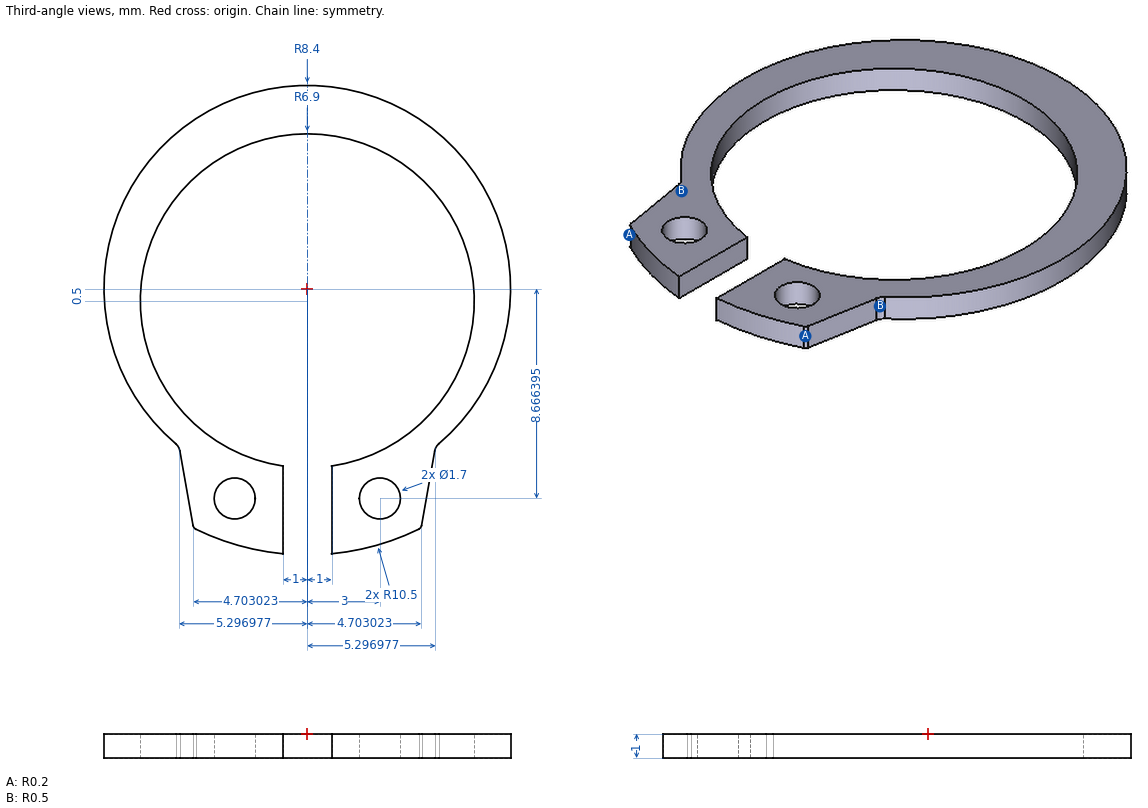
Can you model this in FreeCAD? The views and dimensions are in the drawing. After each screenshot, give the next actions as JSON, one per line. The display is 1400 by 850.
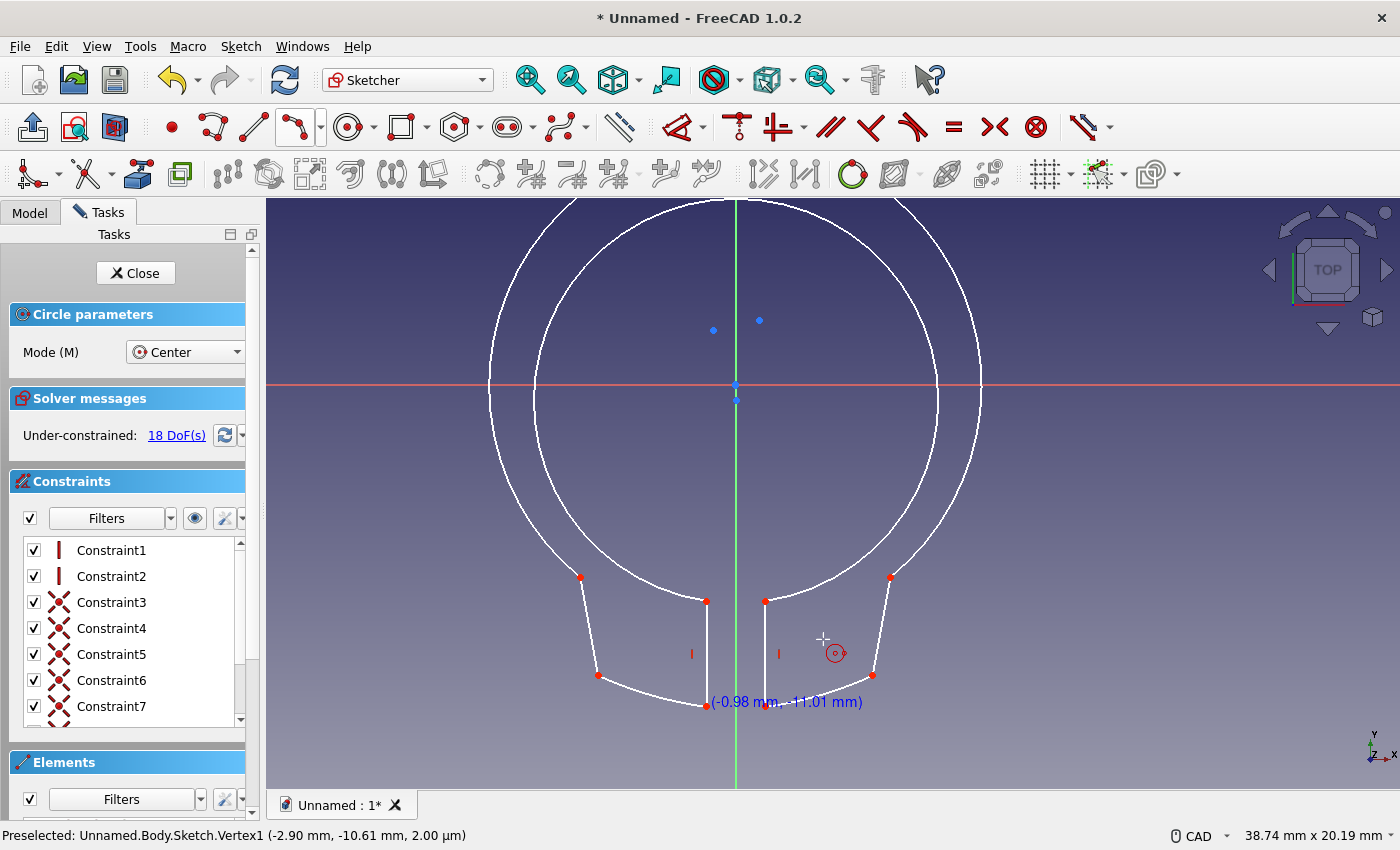
{"action": "left_click", "coordinate": [823, 638]}
{"action": "left_click", "coordinate": [841, 621]}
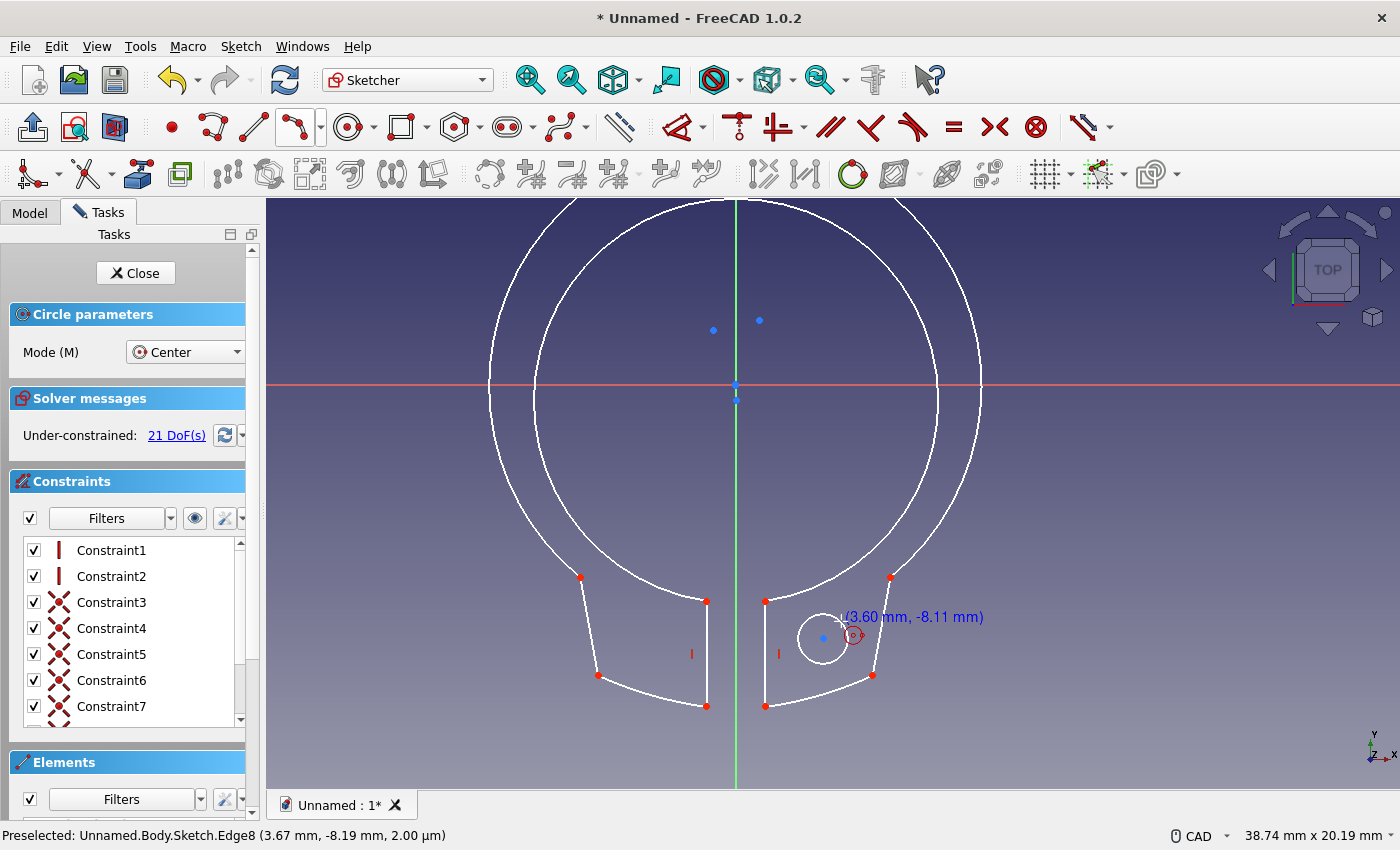
{"action": "left_click", "coordinate": [648, 638]}
{"action": "left_click", "coordinate": [665, 621]}
{"action": "key", "text": "Escape"}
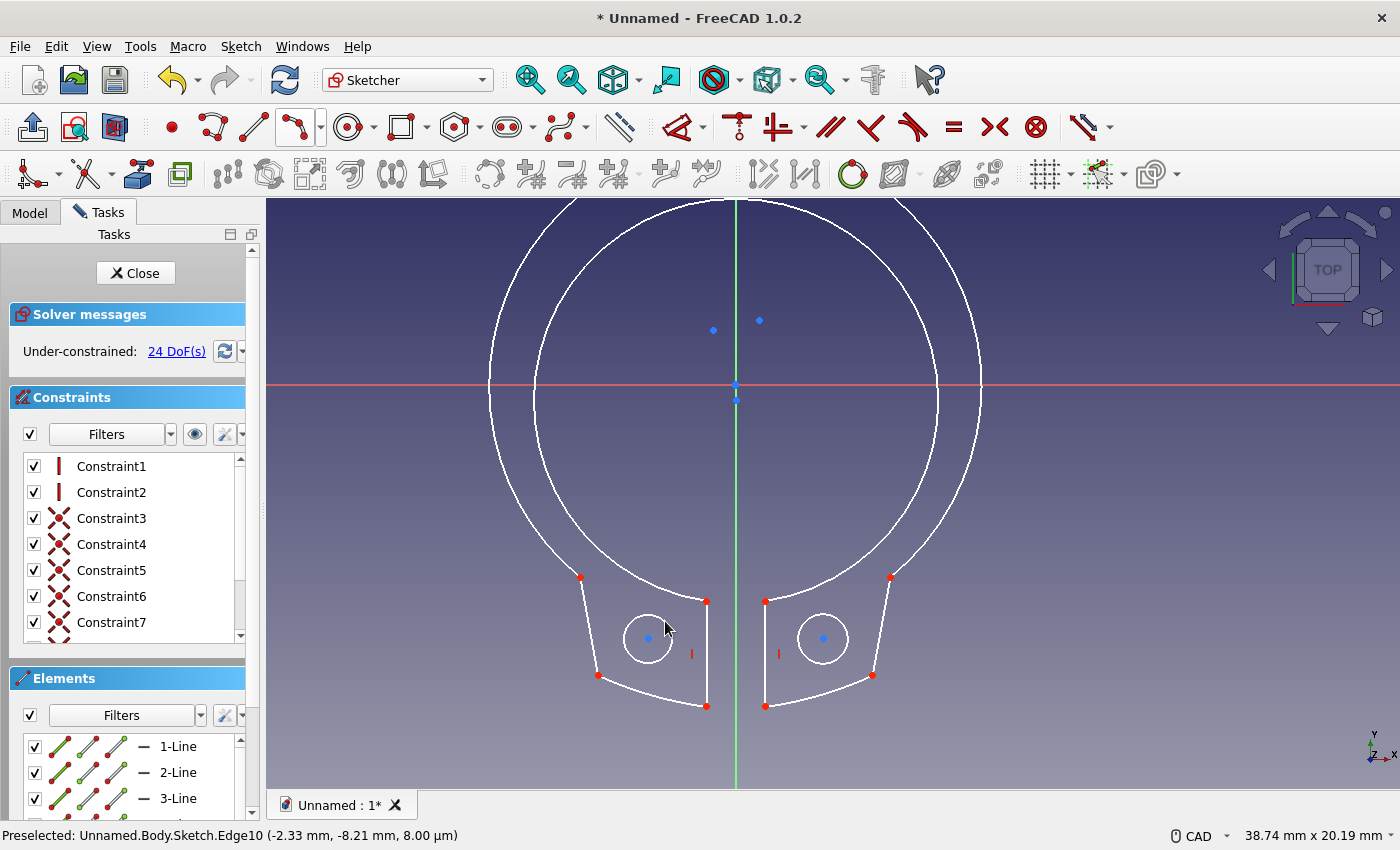
{"action": "left_click", "coordinate": [924, 327]}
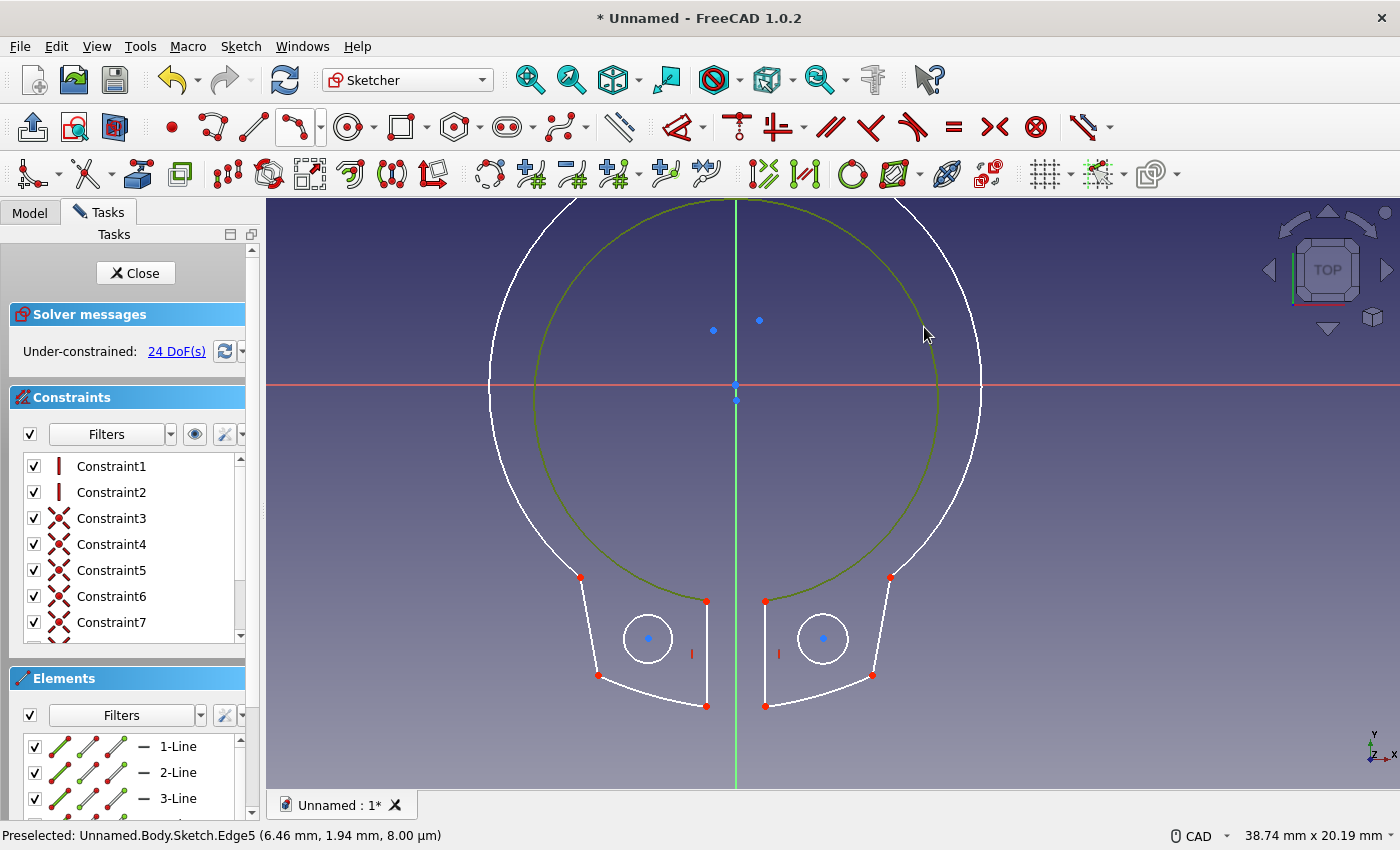
{"action": "left_click", "coordinate": [798, 701]}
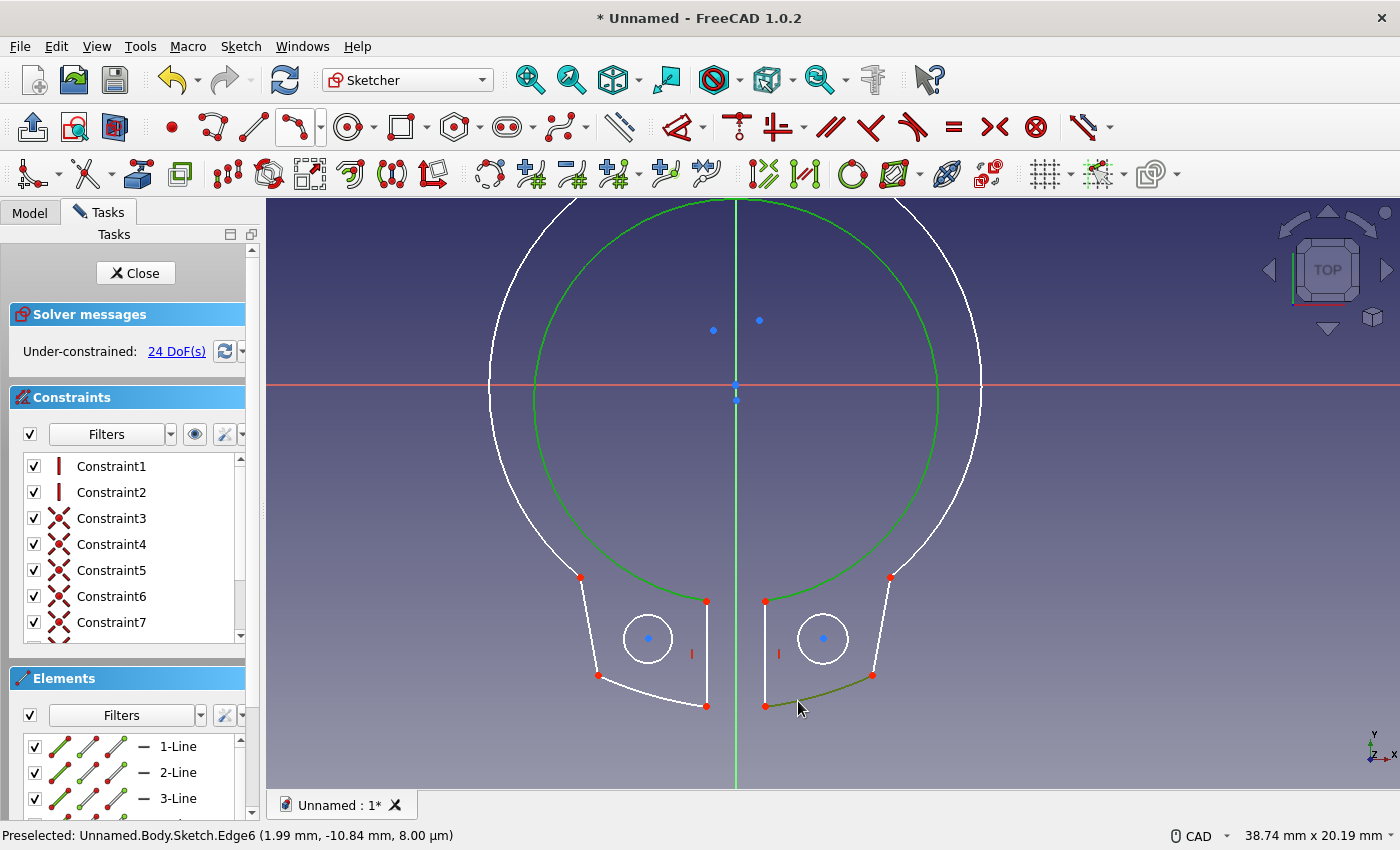
{"action": "left_click", "coordinate": [737, 128]}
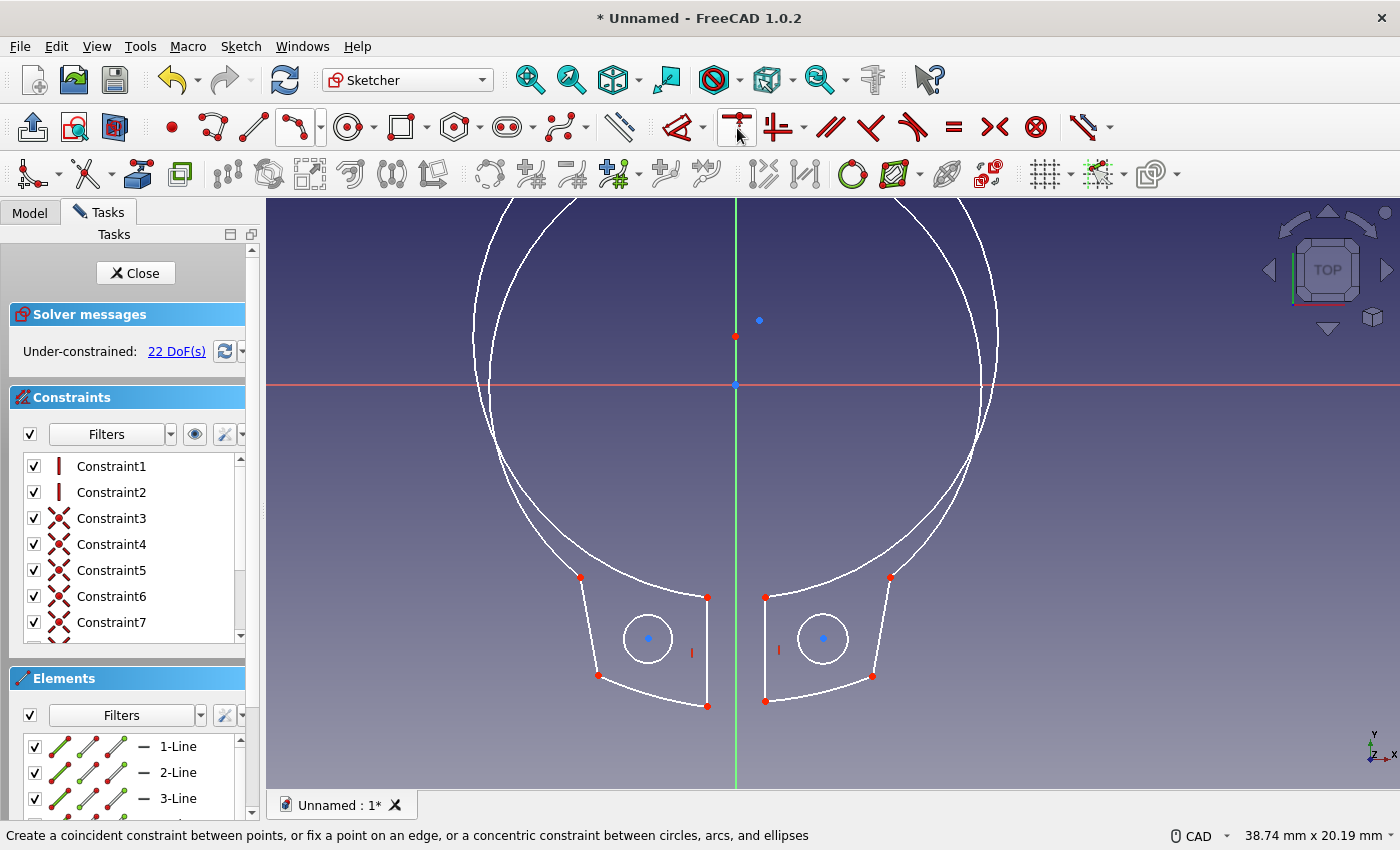
{"action": "left_click", "coordinate": [981, 244]}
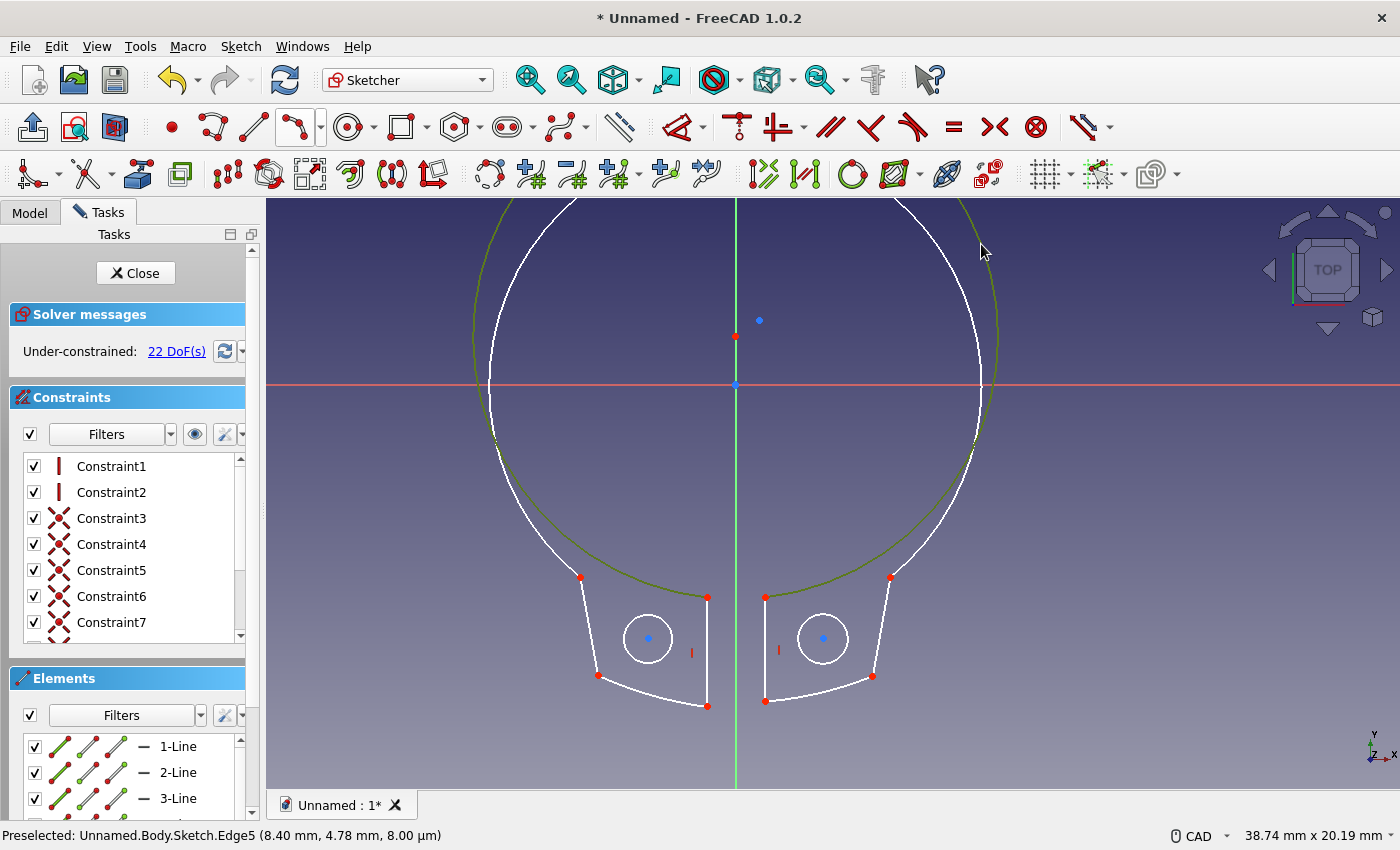
{"action": "left_click", "coordinate": [630, 688]}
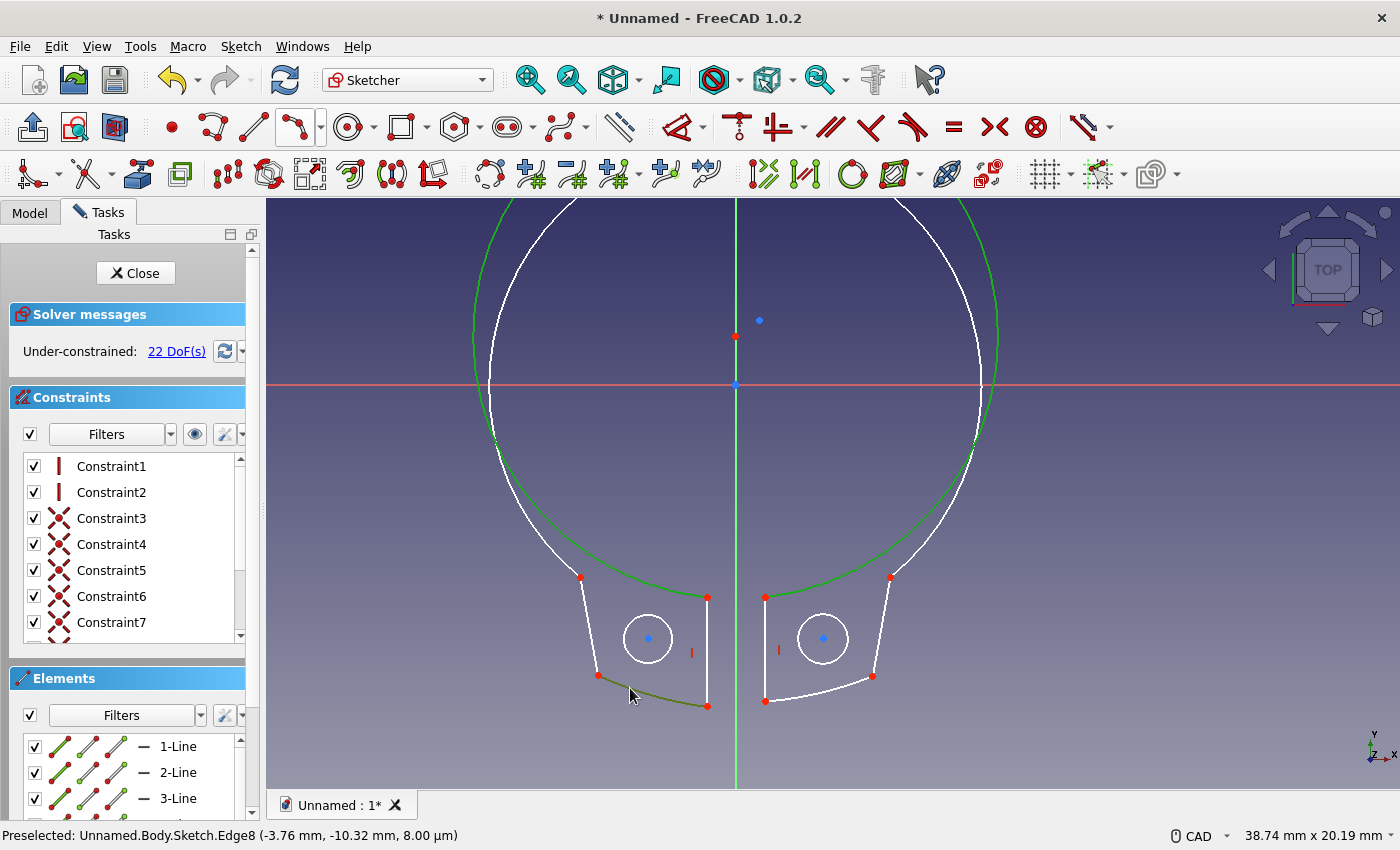
{"action": "left_click", "coordinate": [737, 128]}